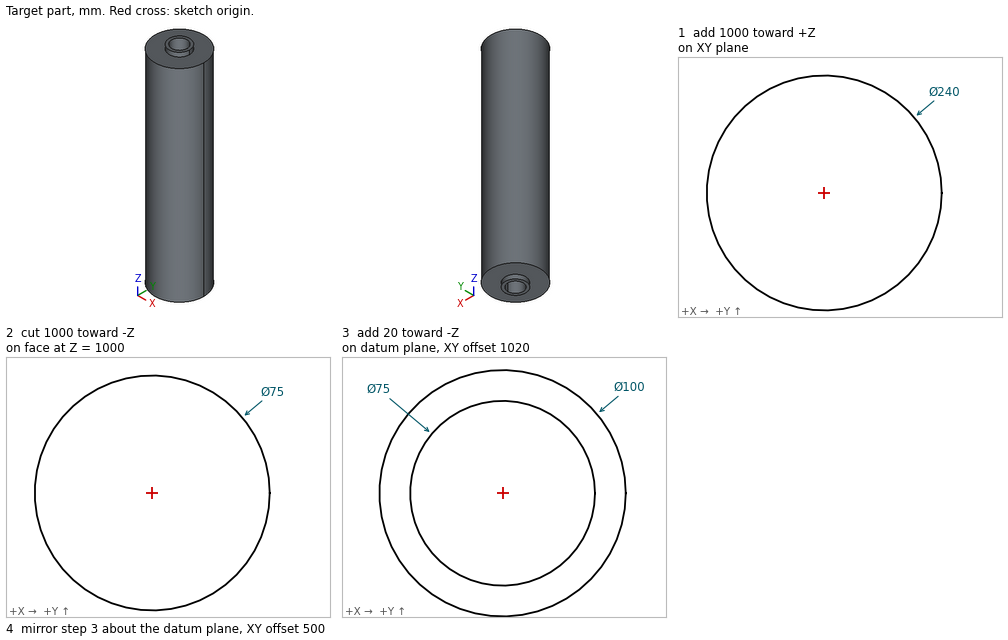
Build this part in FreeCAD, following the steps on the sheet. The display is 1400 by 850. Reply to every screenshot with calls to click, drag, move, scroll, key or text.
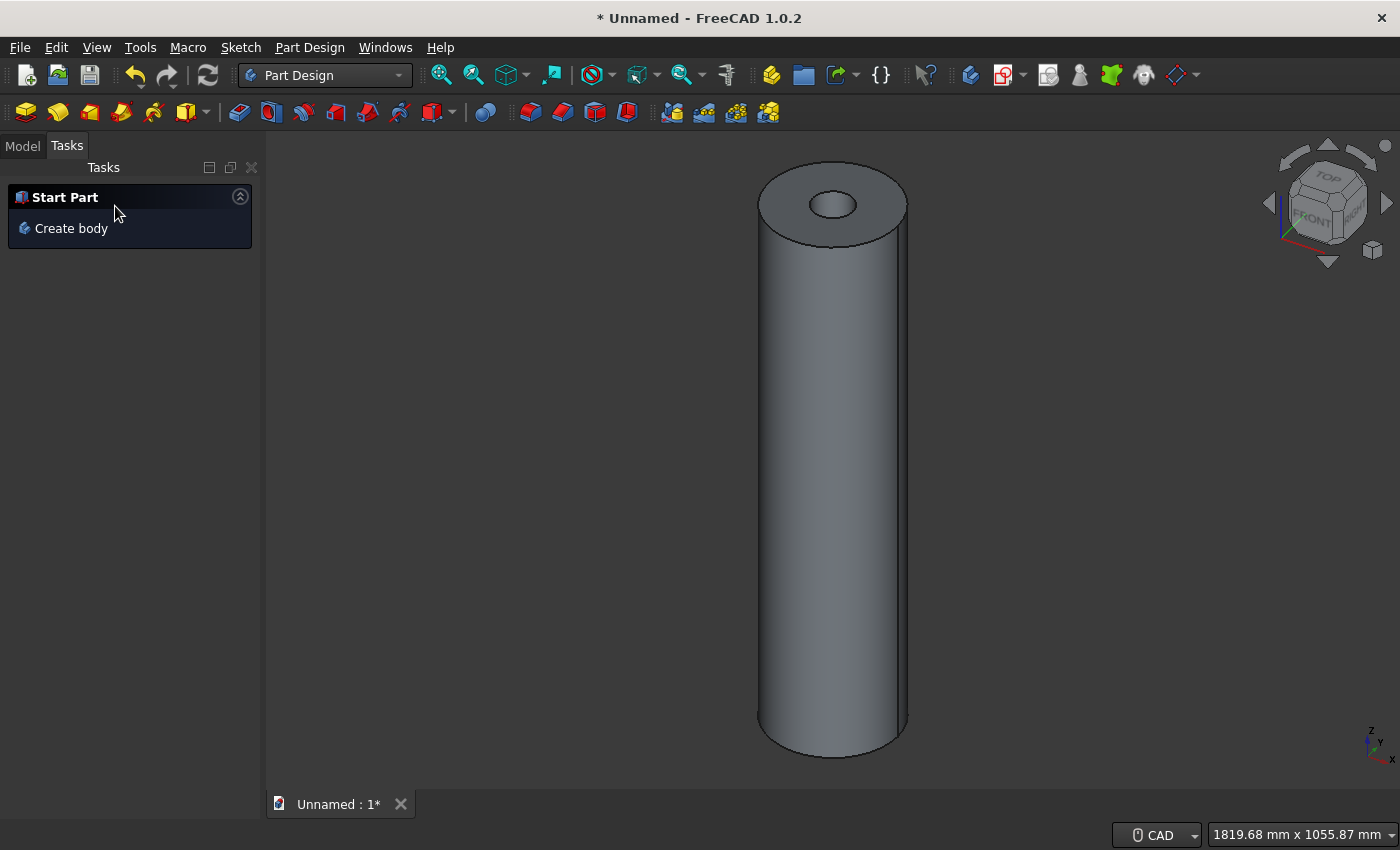
click(23, 145)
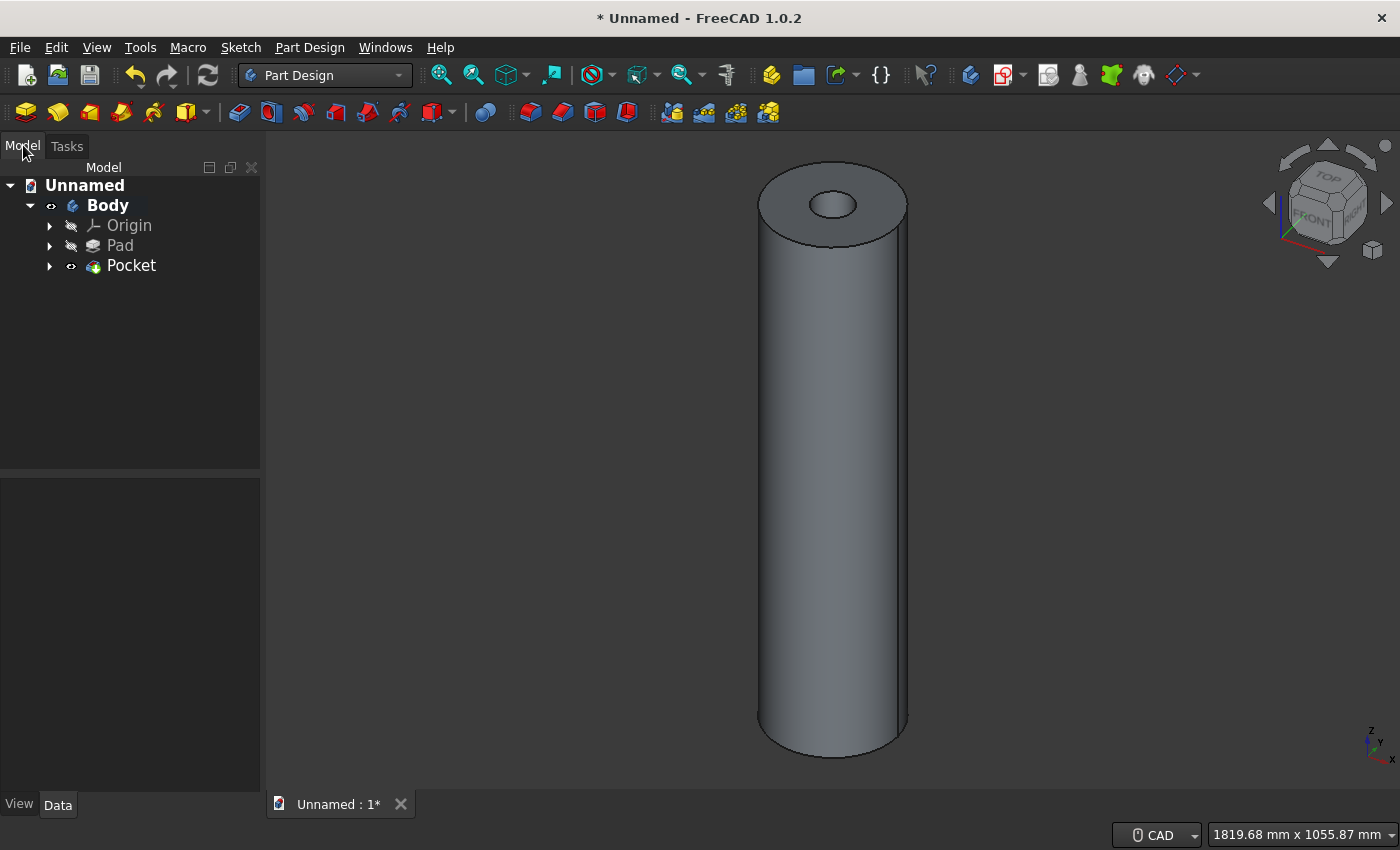
click(50, 226)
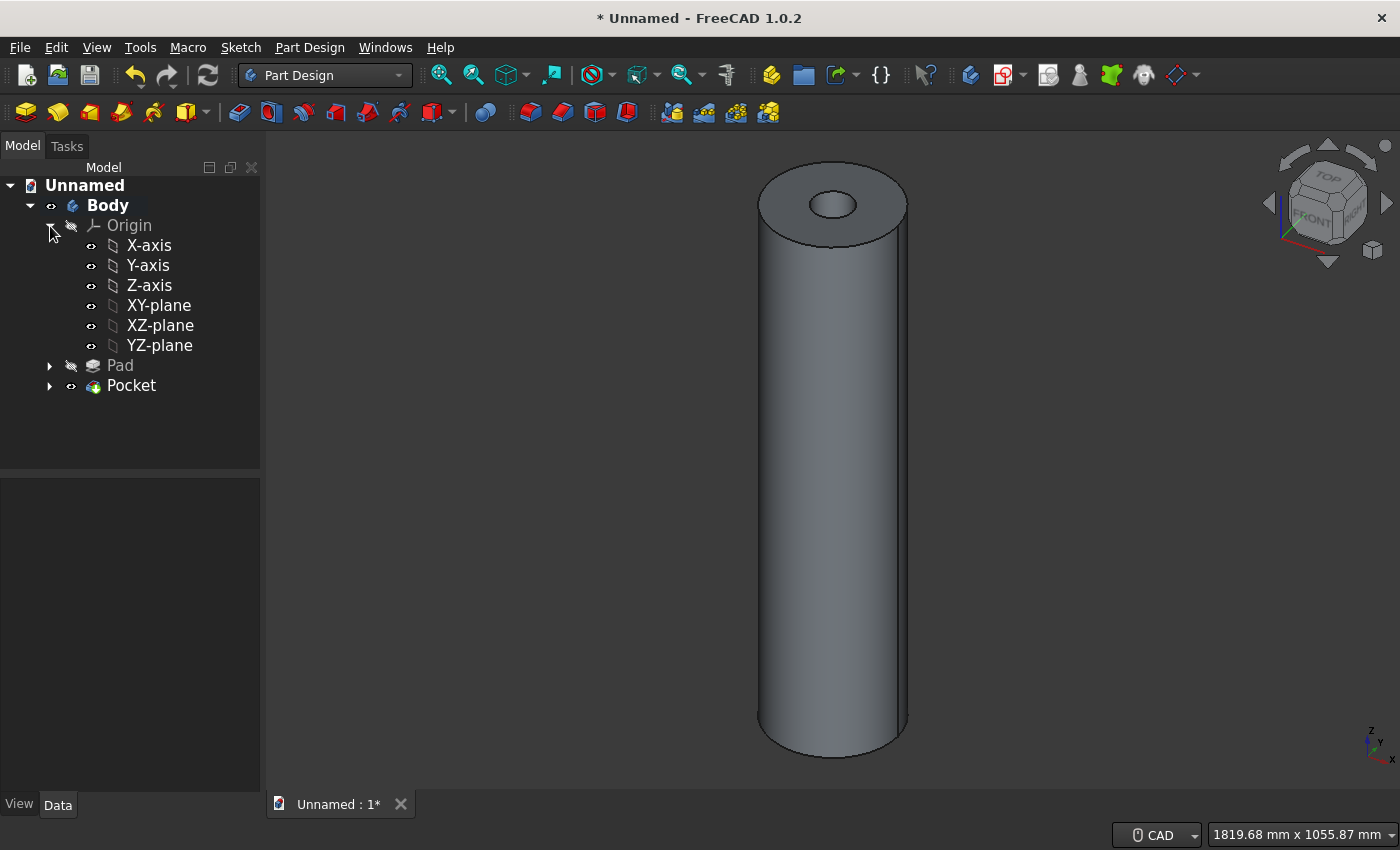
click(136, 306)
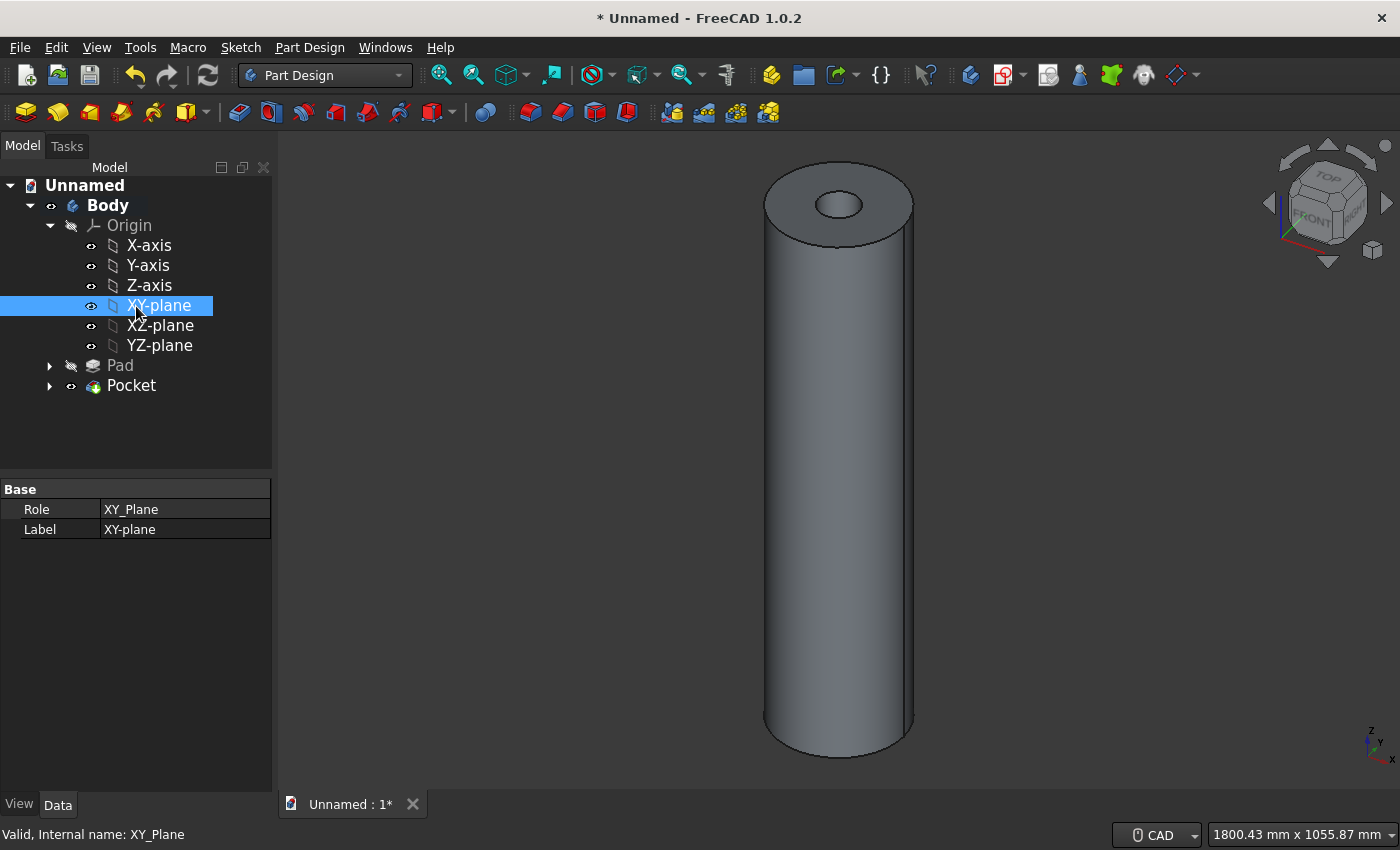
click(1176, 76)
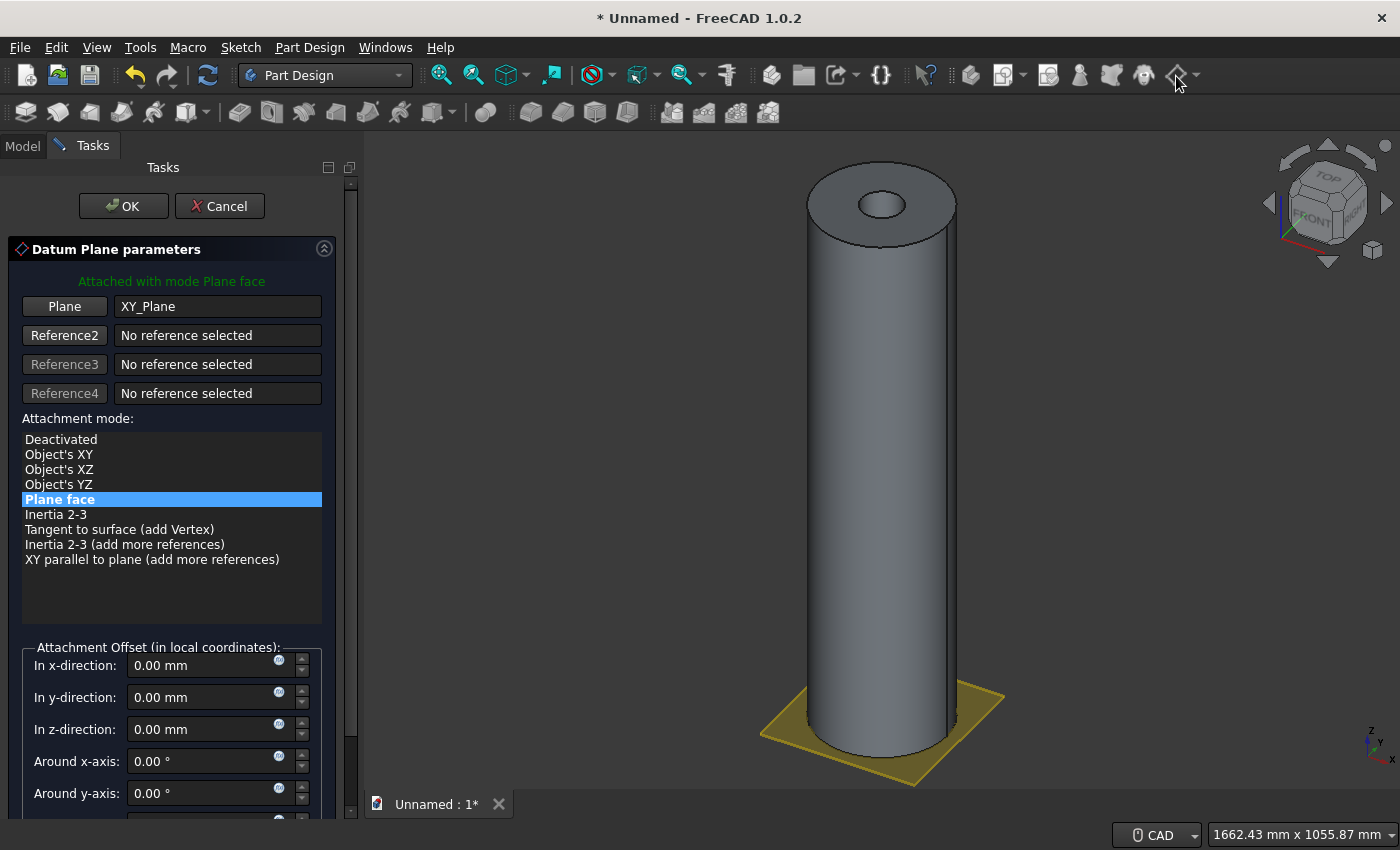
triple_click(210, 729)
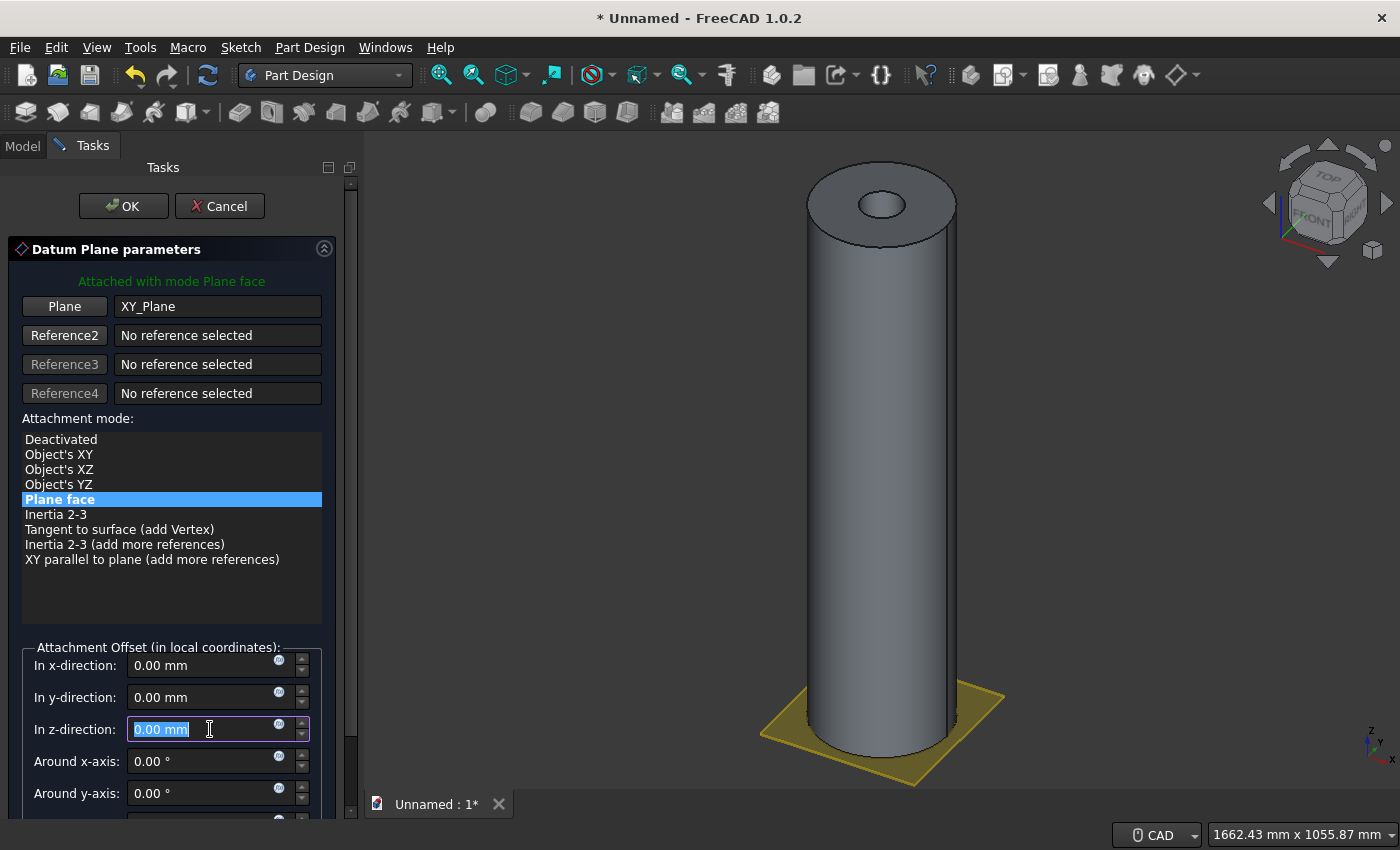
text(1020)
key(Tab)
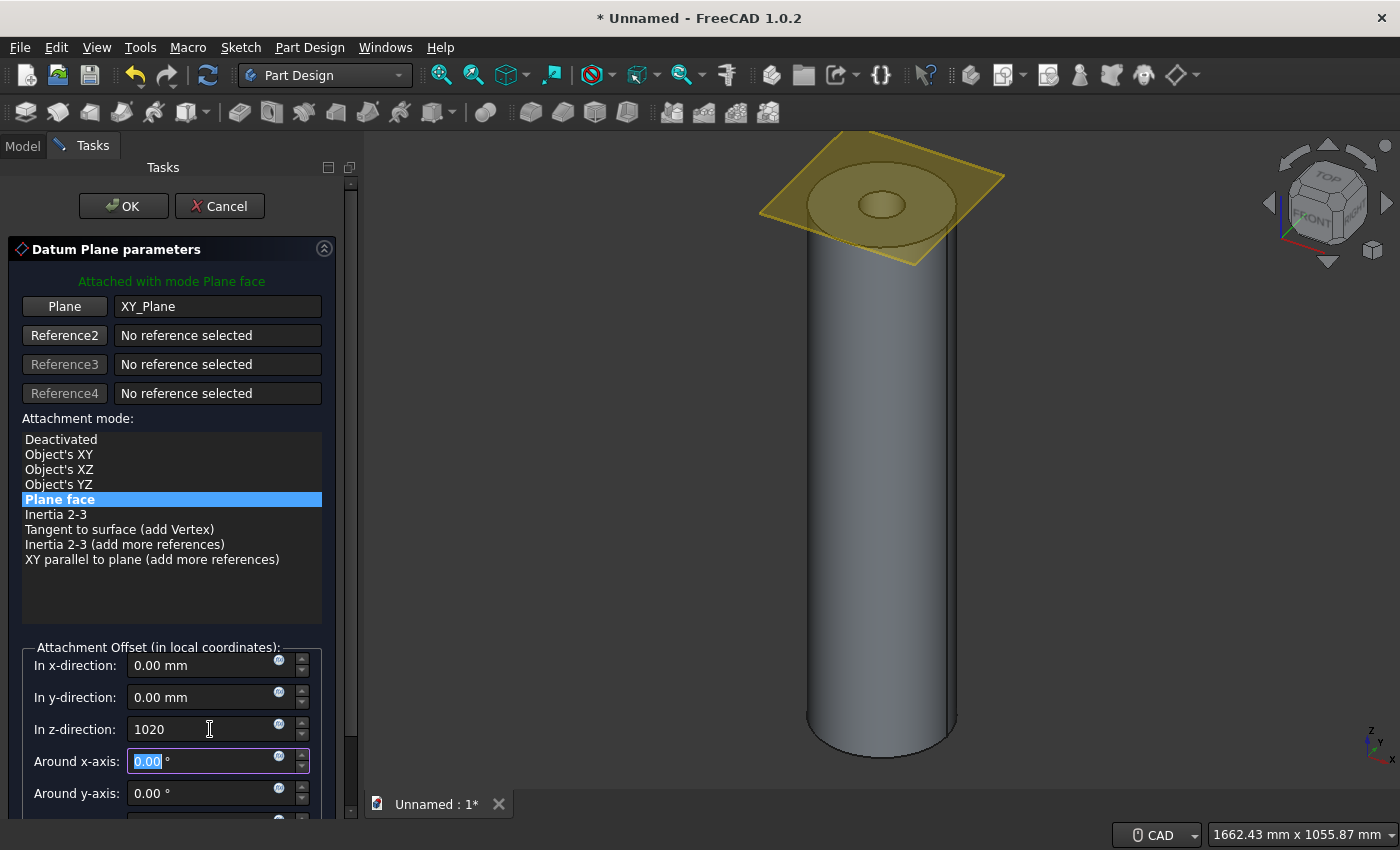
click(124, 206)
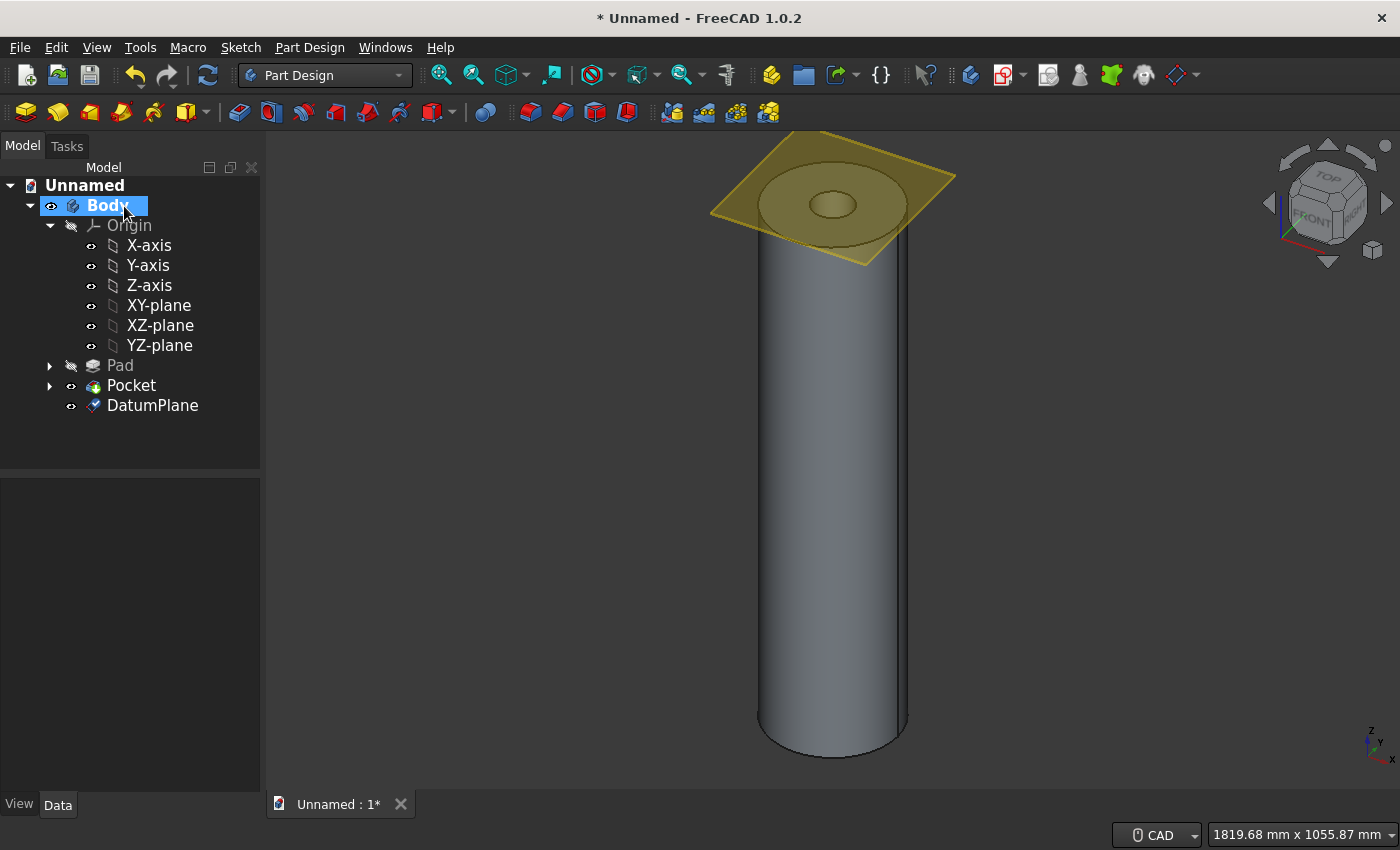
click(116, 406)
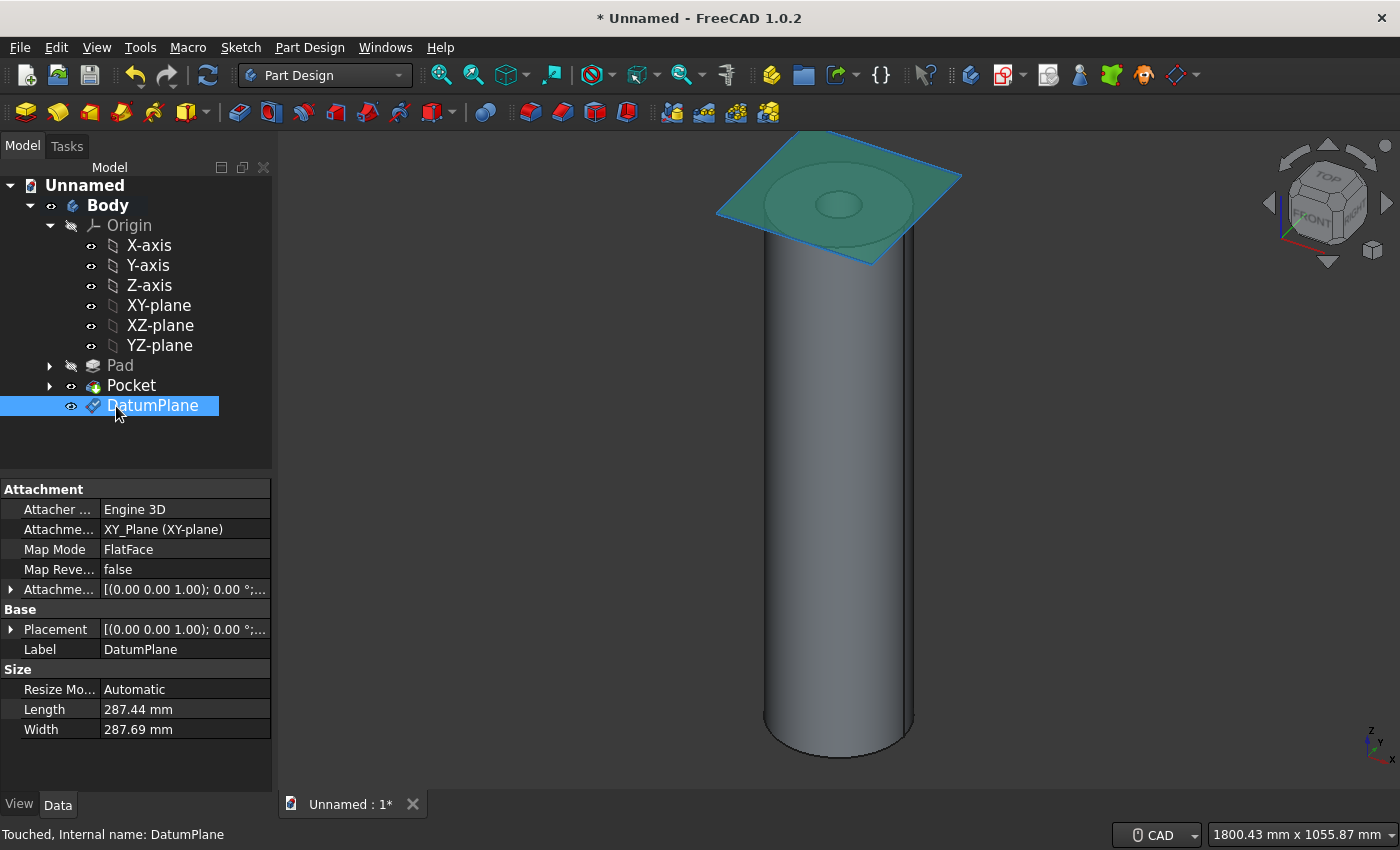
click(1004, 76)